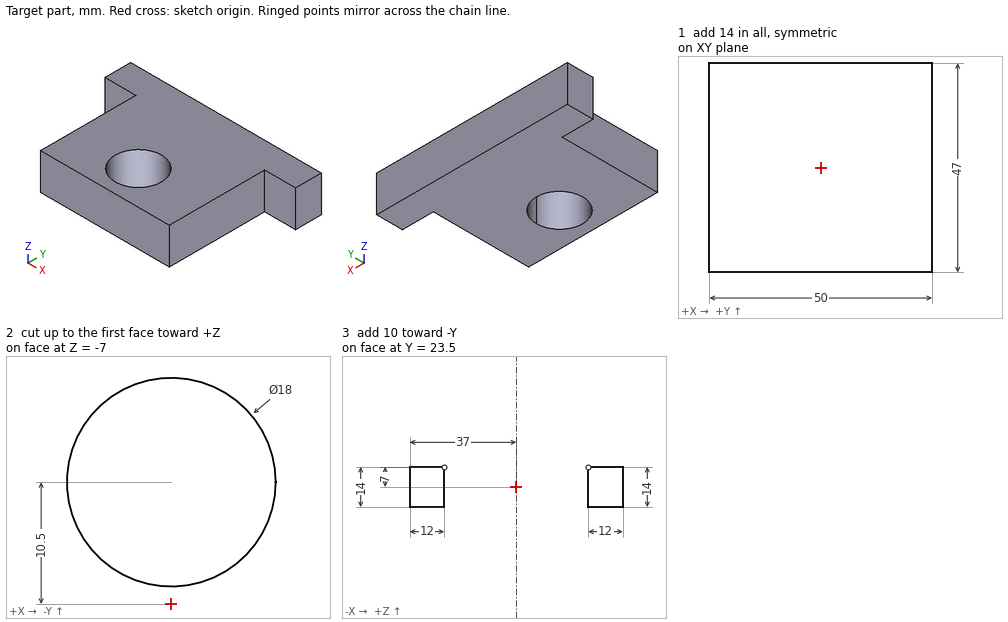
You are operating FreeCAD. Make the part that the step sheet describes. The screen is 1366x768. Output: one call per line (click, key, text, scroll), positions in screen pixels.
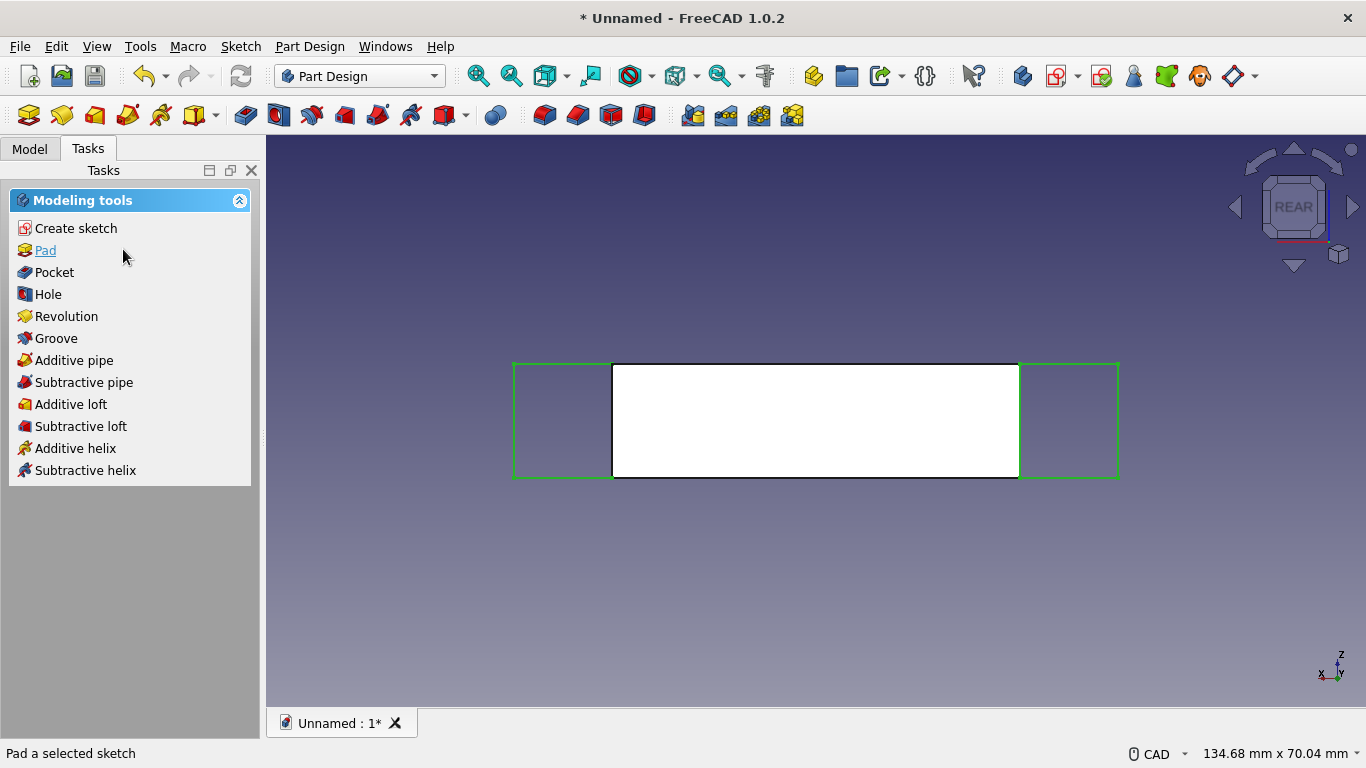
click(29, 116)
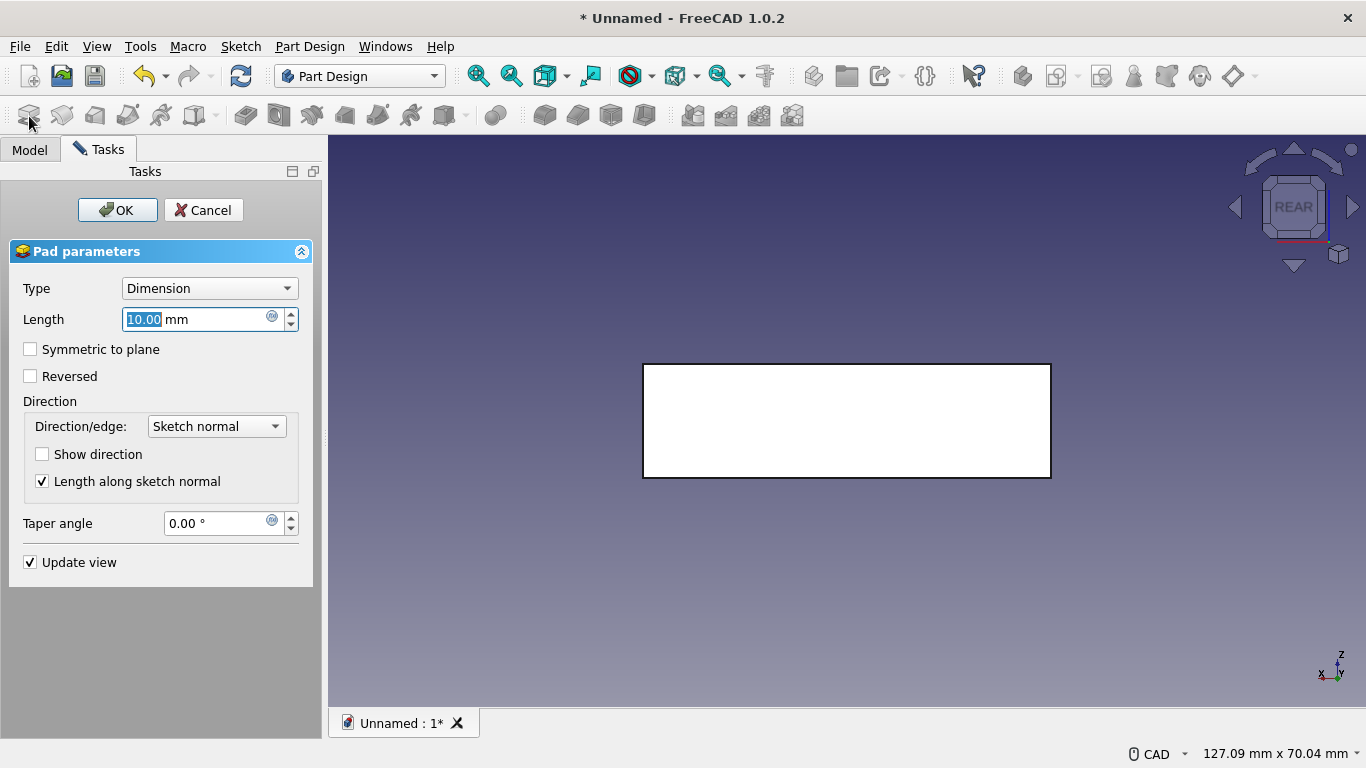
text(10)
key(Tab)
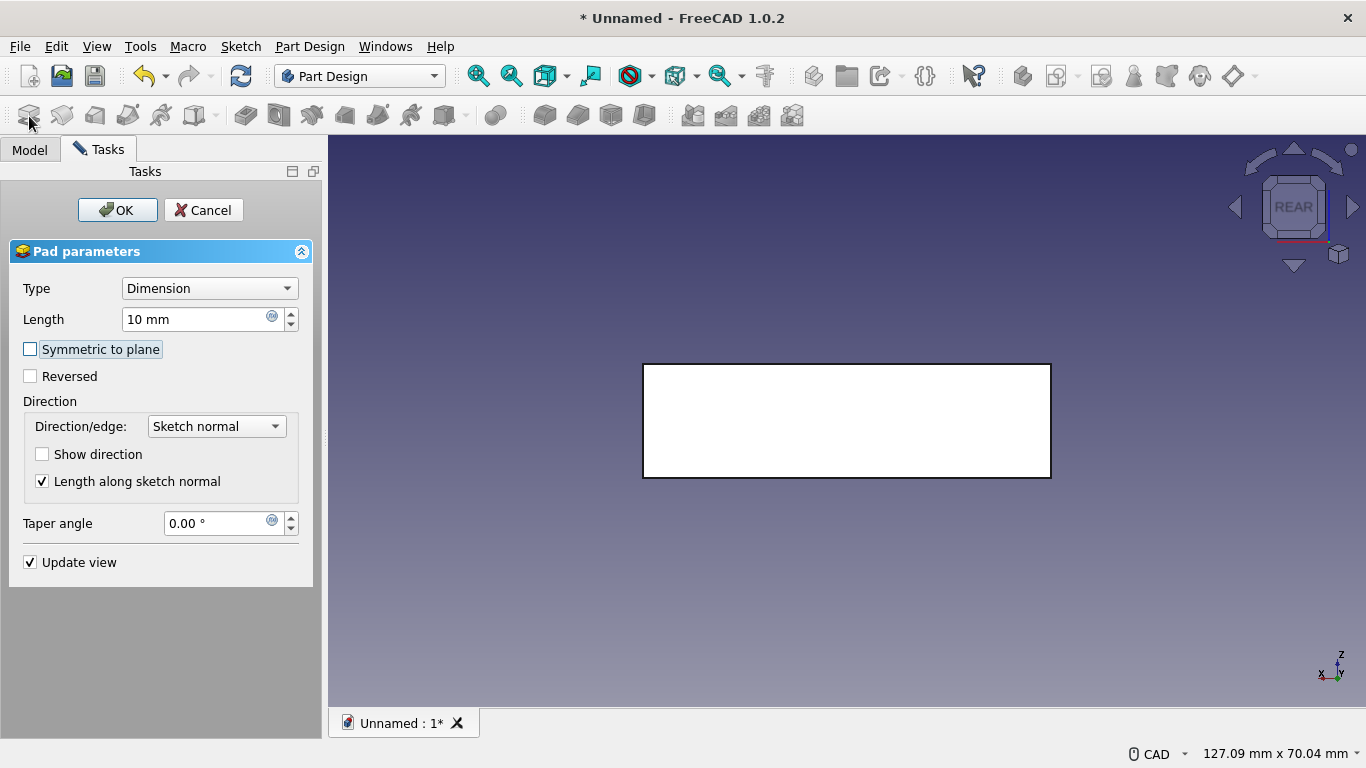
click(31, 376)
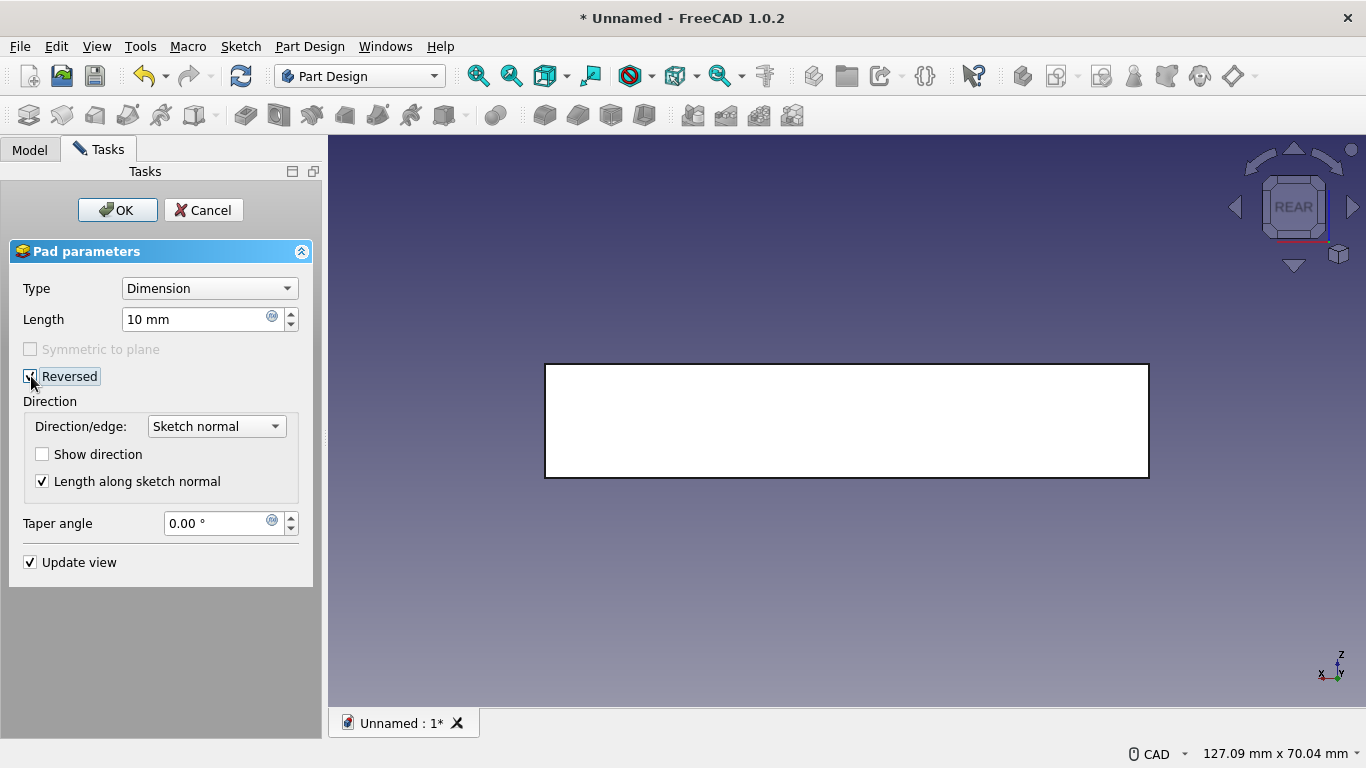
click(118, 210)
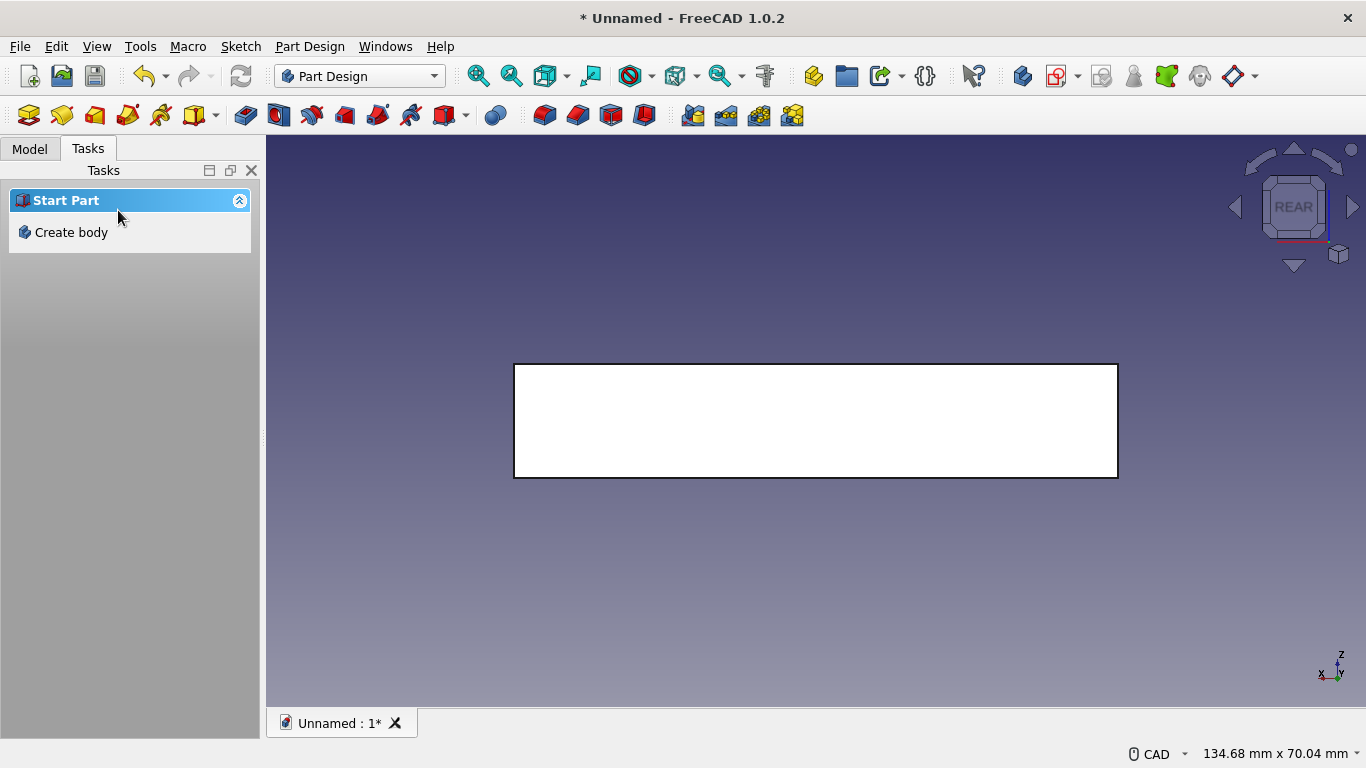
key(0)